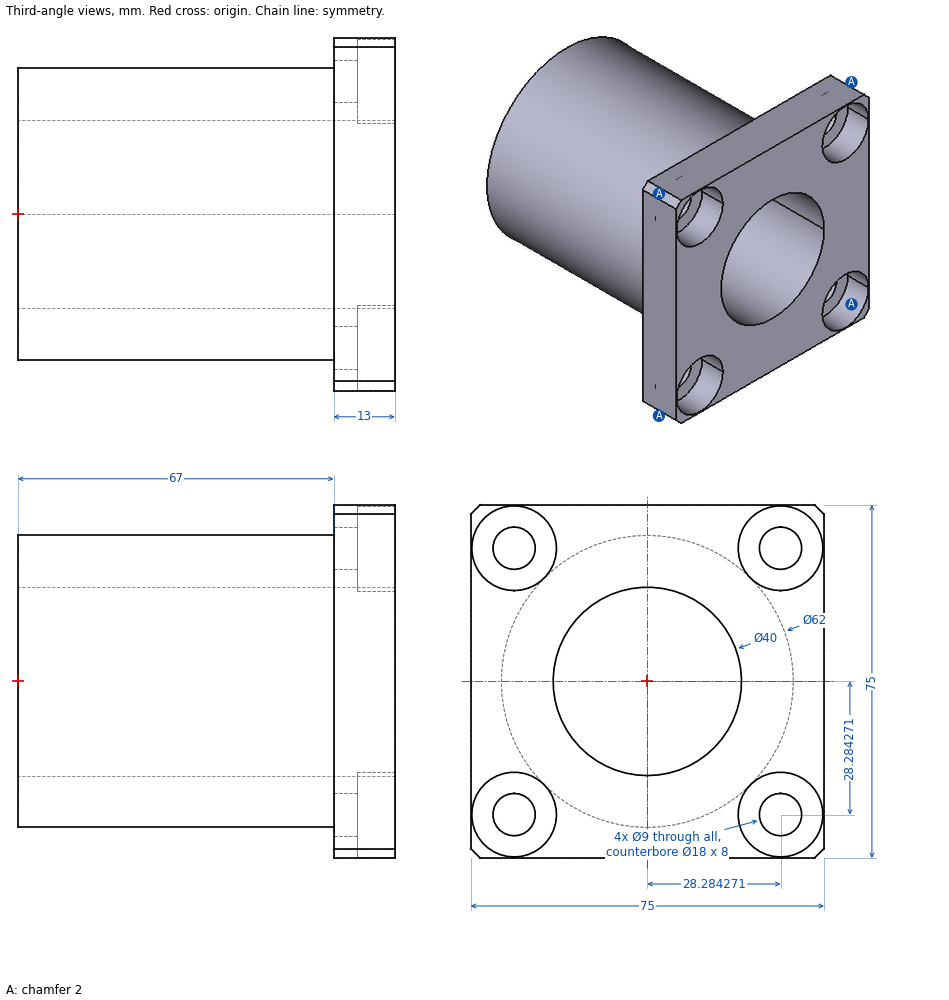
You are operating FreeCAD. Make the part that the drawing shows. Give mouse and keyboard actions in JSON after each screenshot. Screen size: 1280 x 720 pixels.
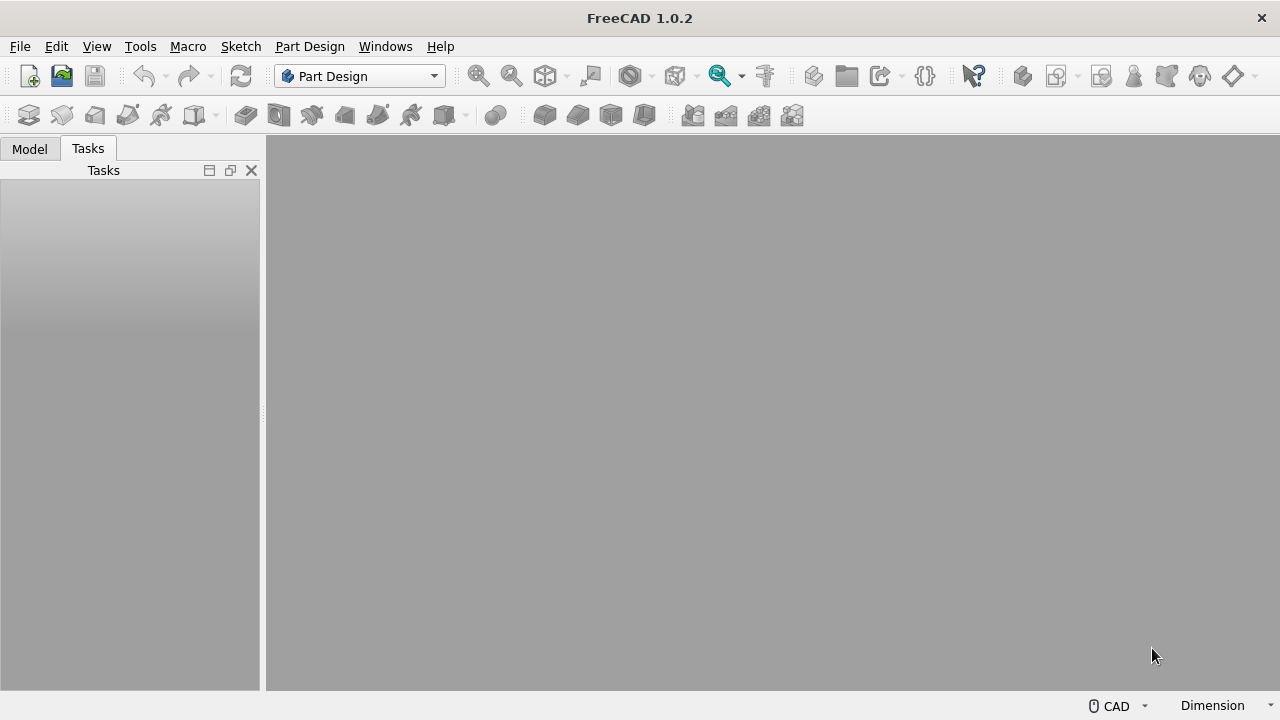
{"action": "left_click", "coordinate": [29, 76]}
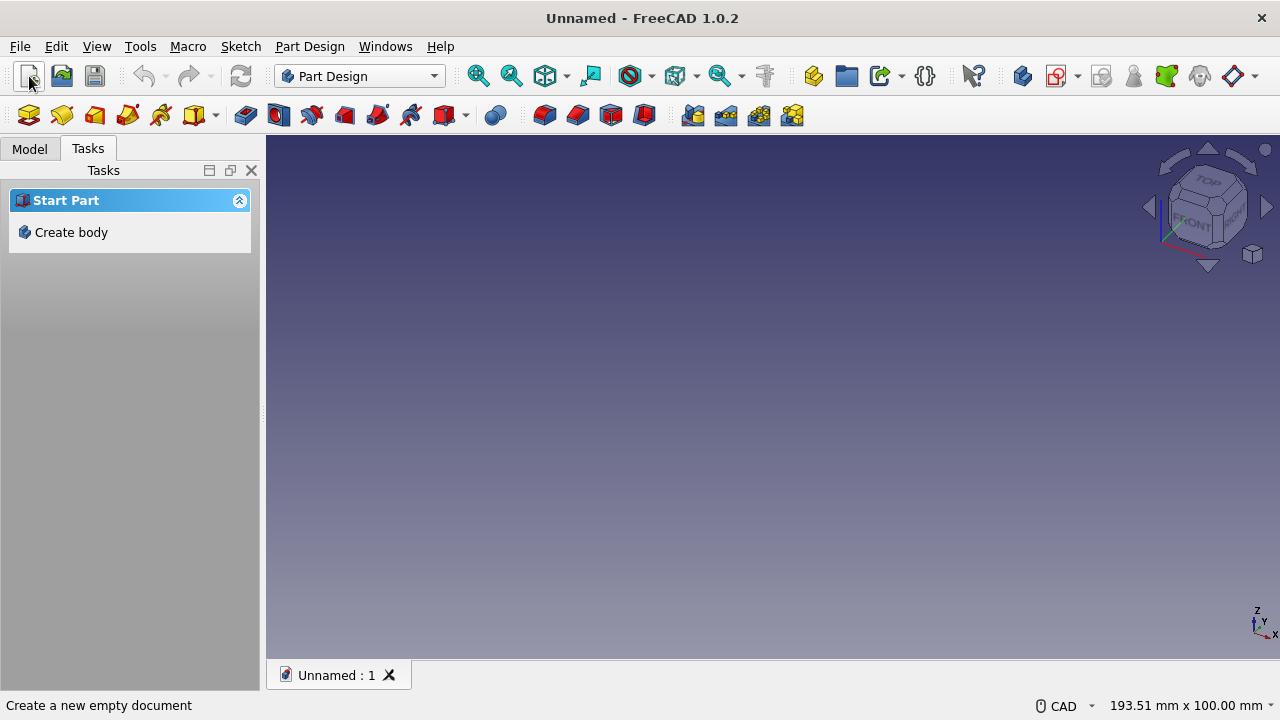
{"action": "left_click", "coordinate": [1056, 76]}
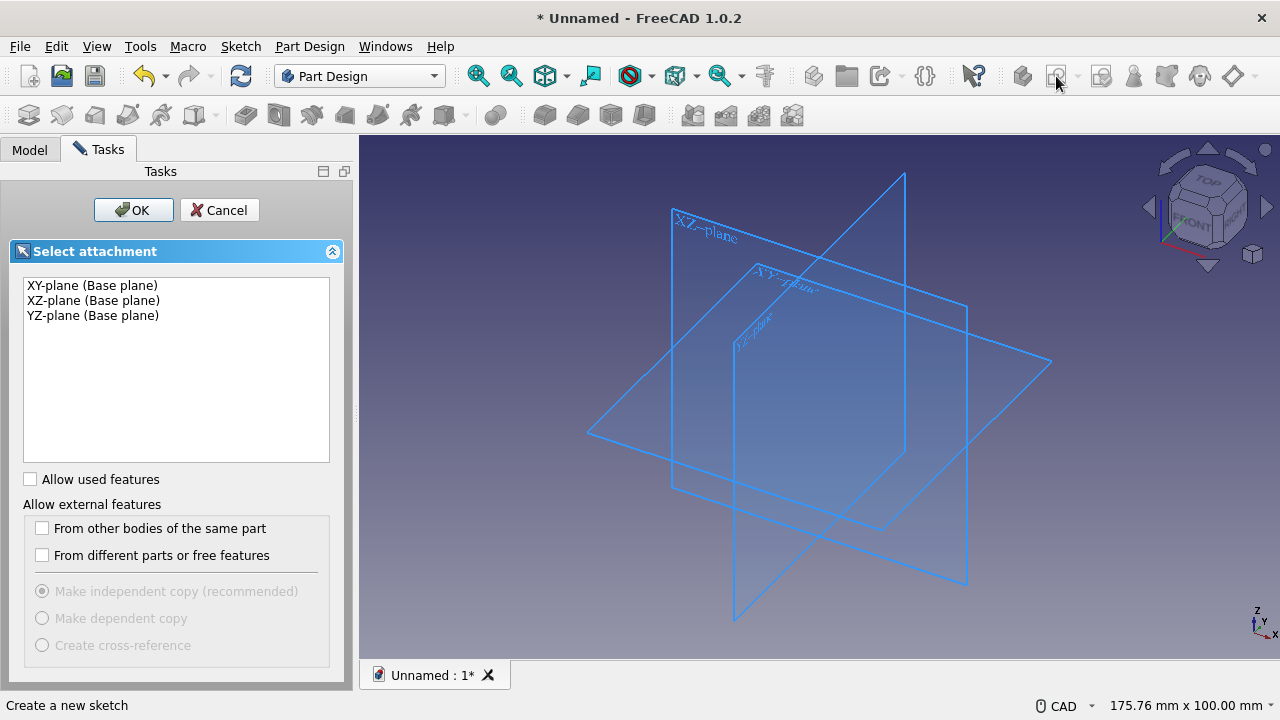
{"action": "left_click", "coordinate": [84, 316]}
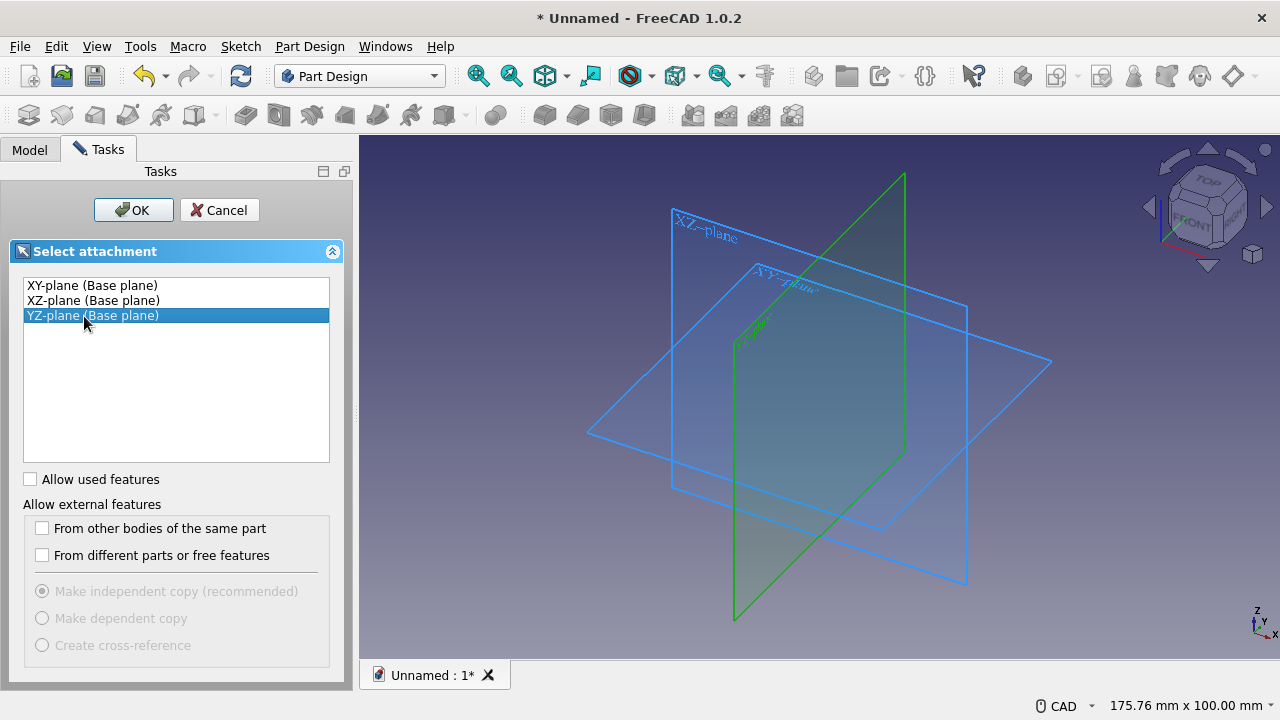
{"action": "left_click", "coordinate": [134, 210]}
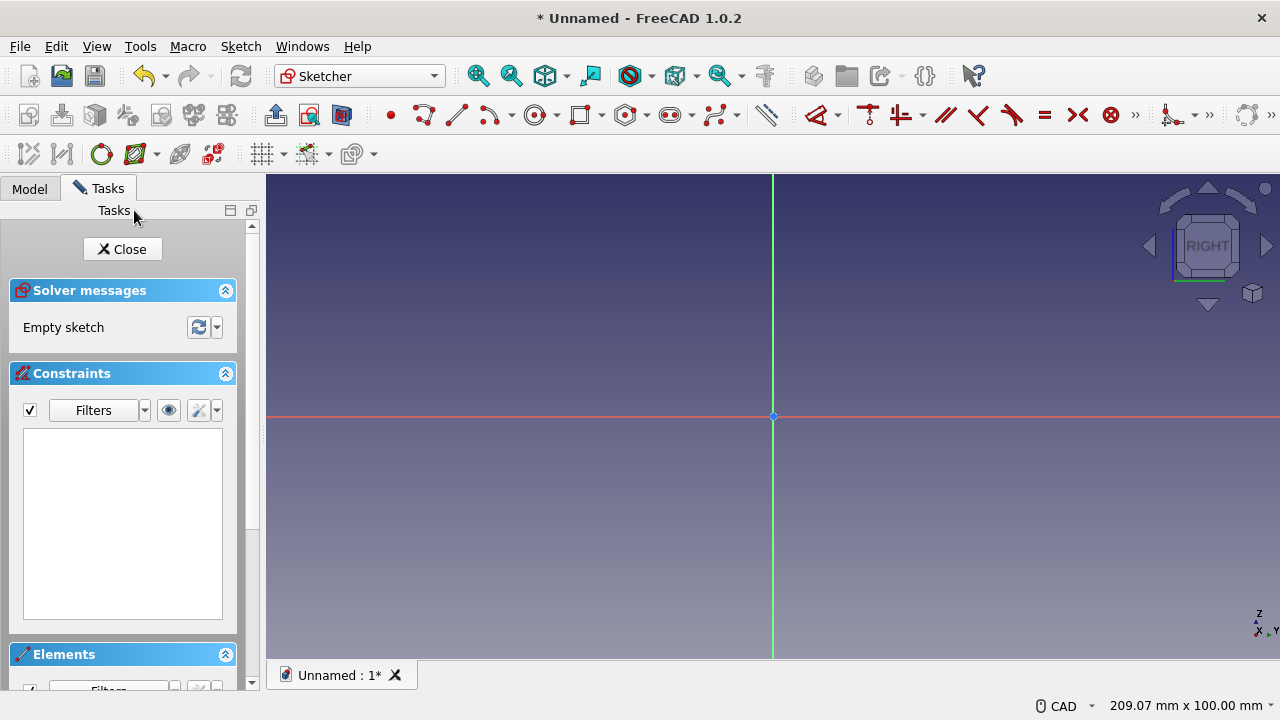
{"action": "left_click", "coordinate": [534, 116]}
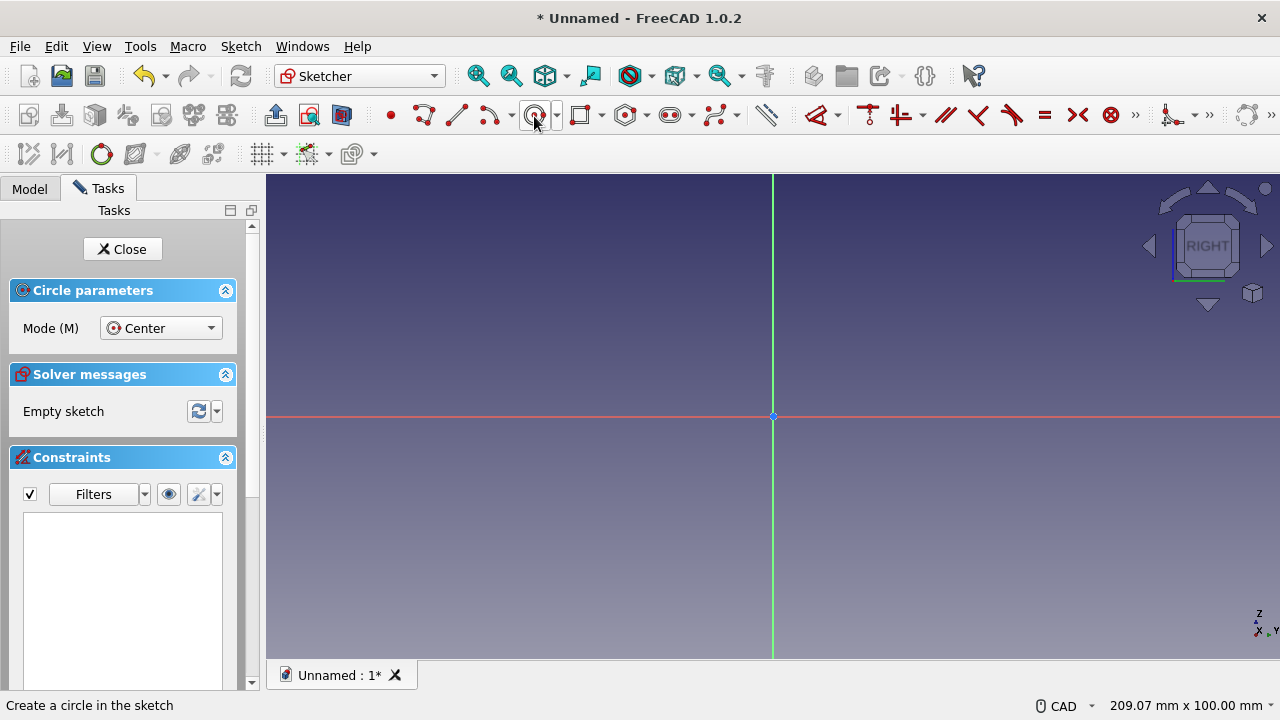
{"action": "left_click", "coordinate": [773, 416]}
{"action": "left_click", "coordinate": [879, 310]}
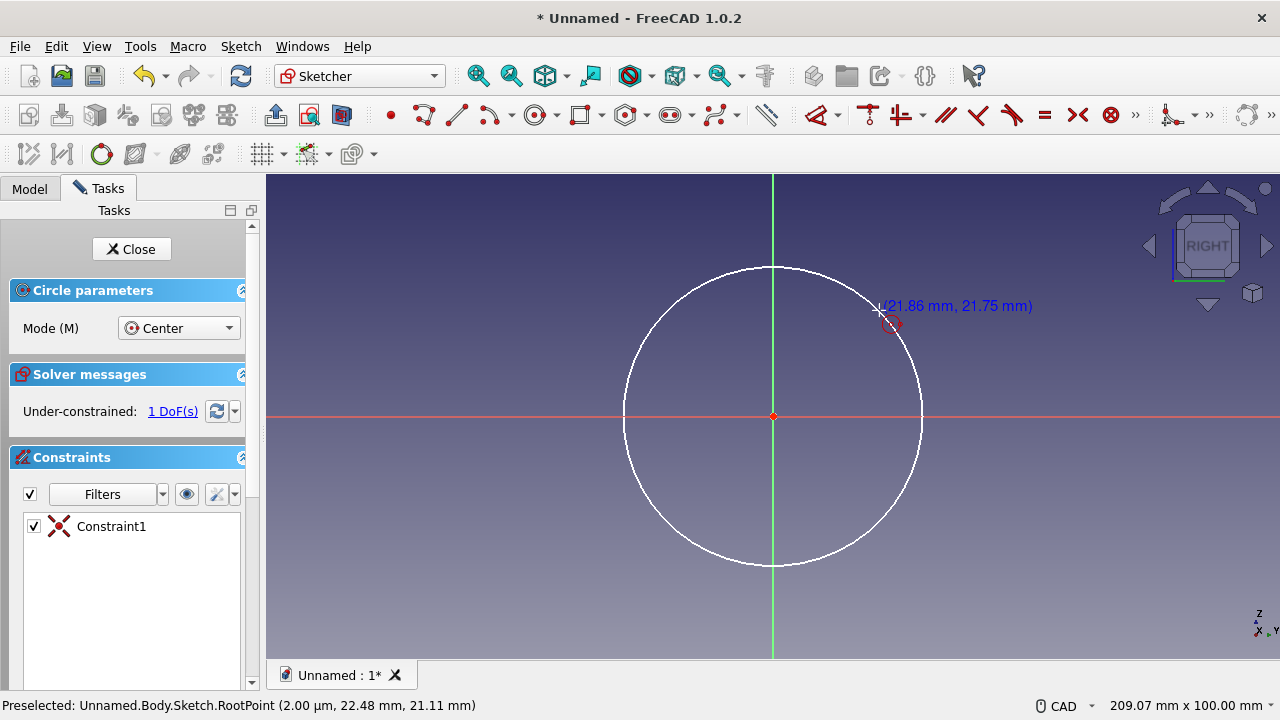
{"action": "left_click", "coordinate": [773, 416]}
{"action": "left_click", "coordinate": [842, 348]}
{"action": "key", "text": "Escape"}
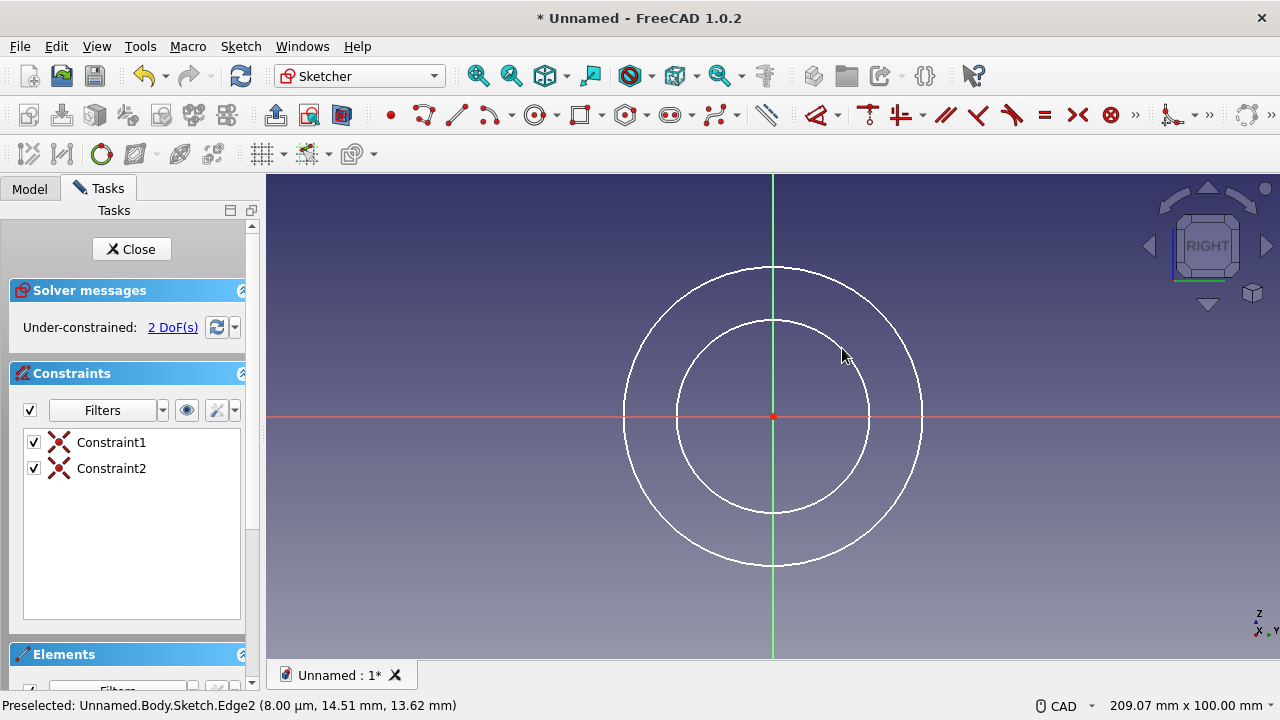
{"action": "left_click", "coordinate": [878, 310]}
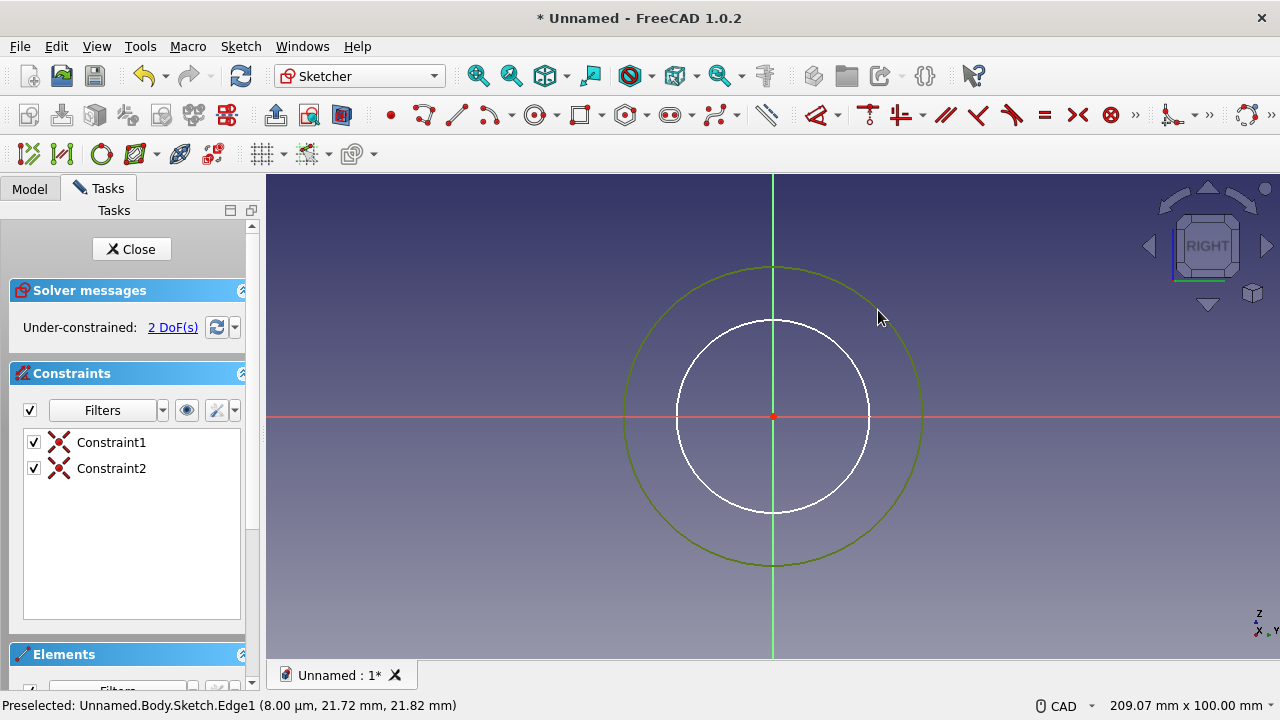
{"action": "left_click", "coordinate": [838, 116]}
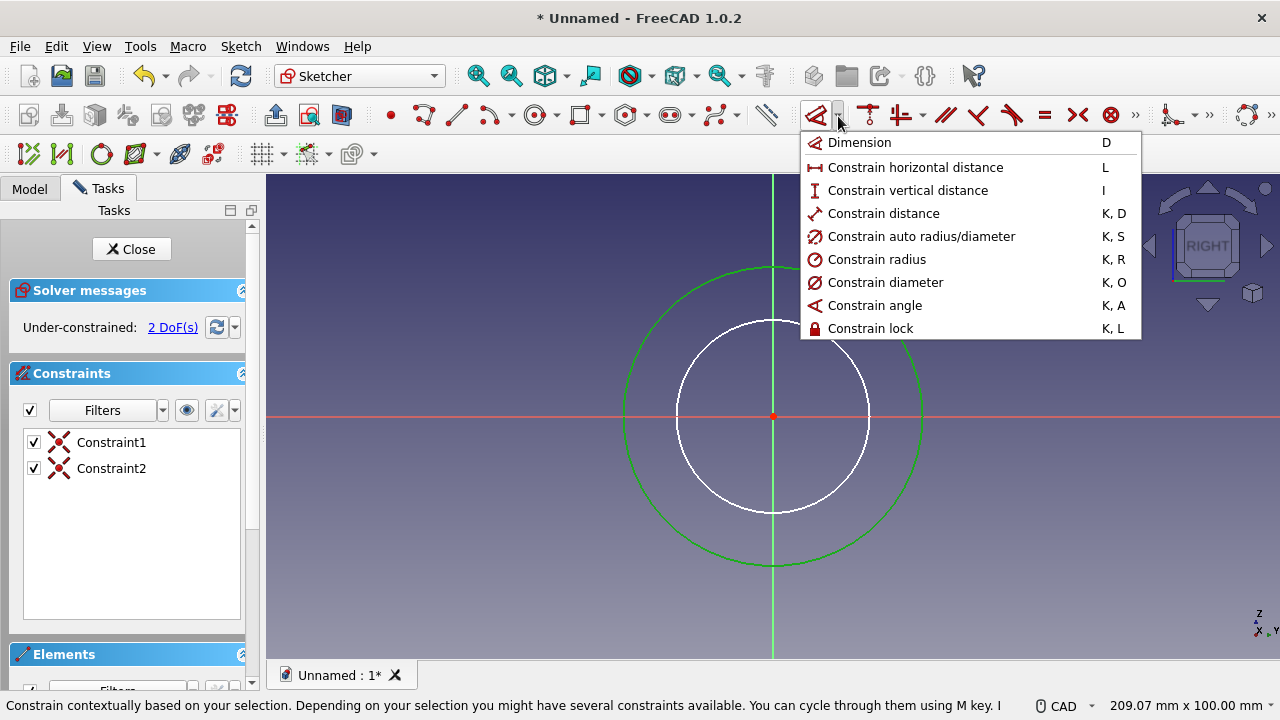
{"action": "left_click", "coordinate": [971, 282]}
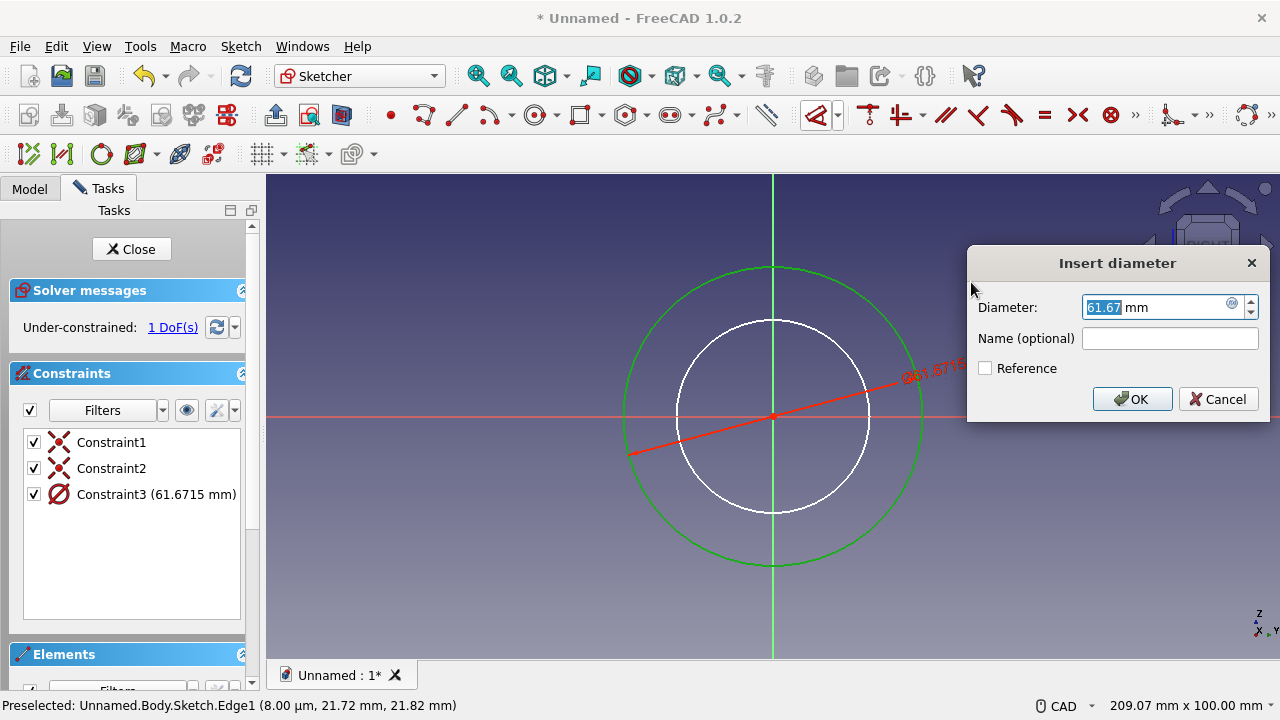
{"action": "type", "text": "62"}
{"action": "key", "text": "Return"}